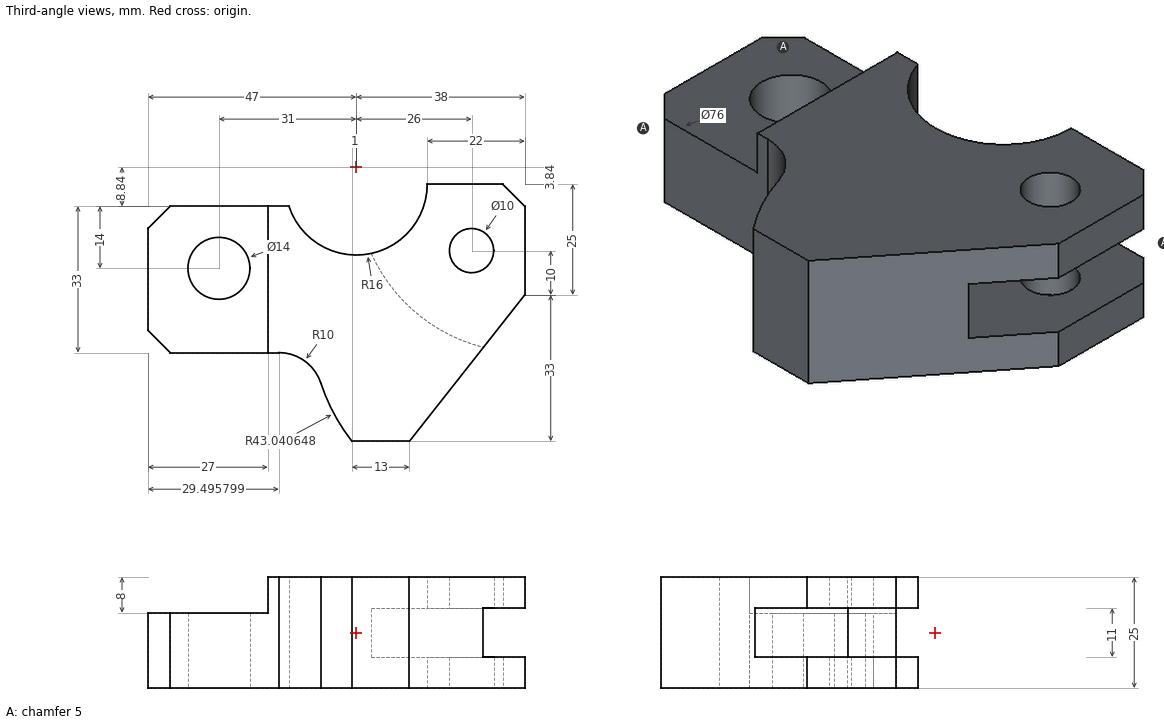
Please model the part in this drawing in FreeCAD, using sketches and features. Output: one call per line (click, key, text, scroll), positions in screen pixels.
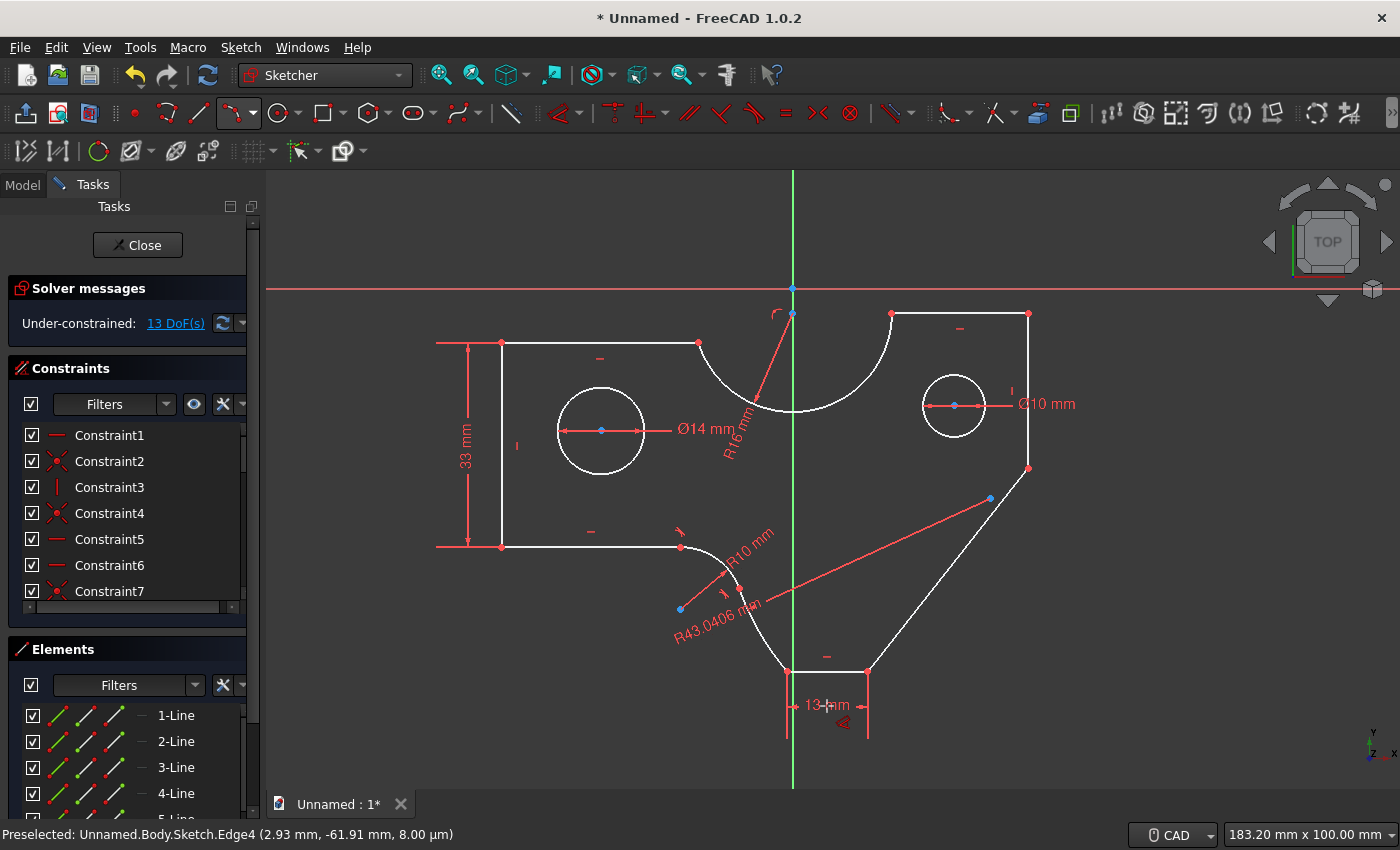
click(1028, 422)
click(1062, 391)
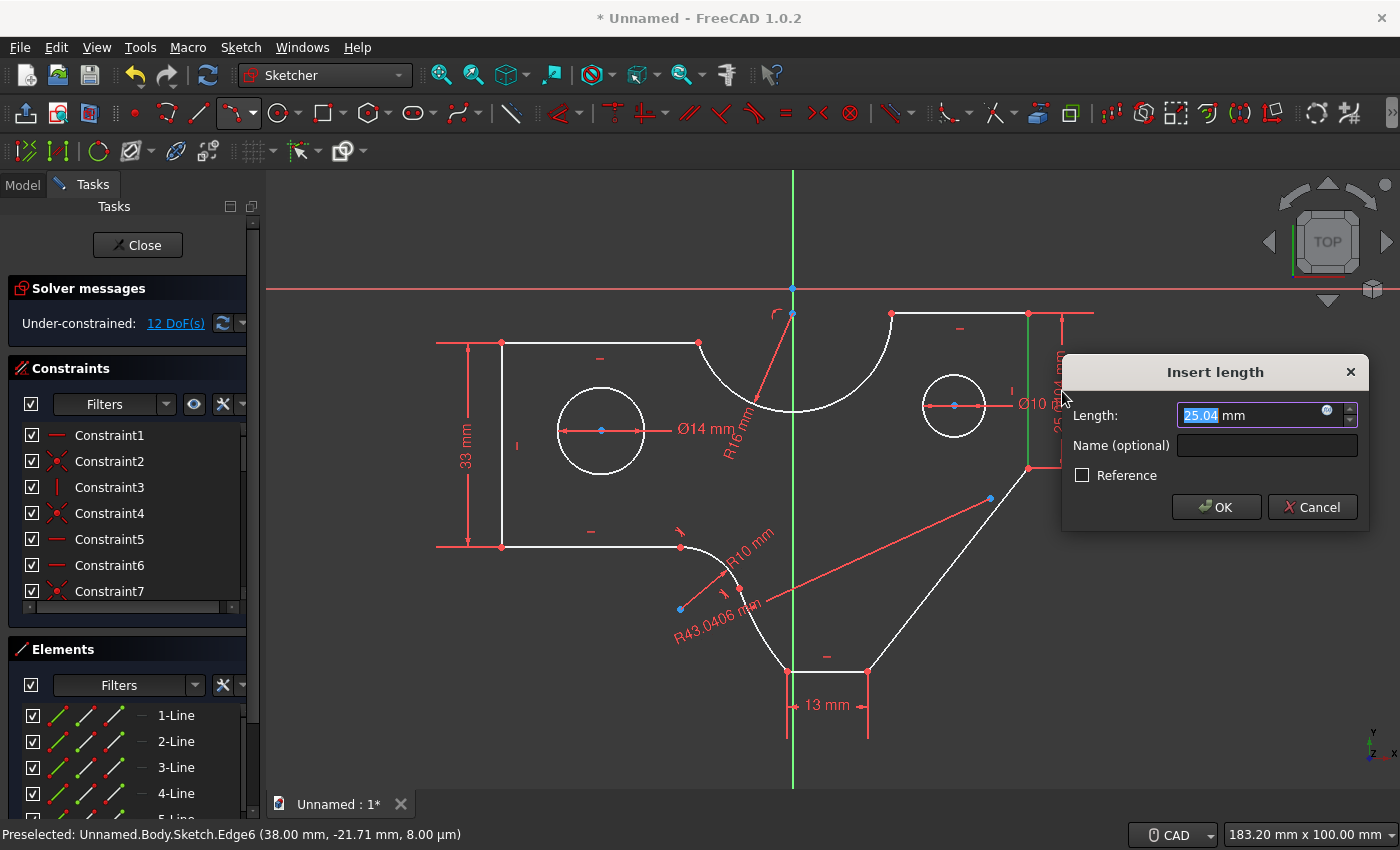
text(25)
key(Return)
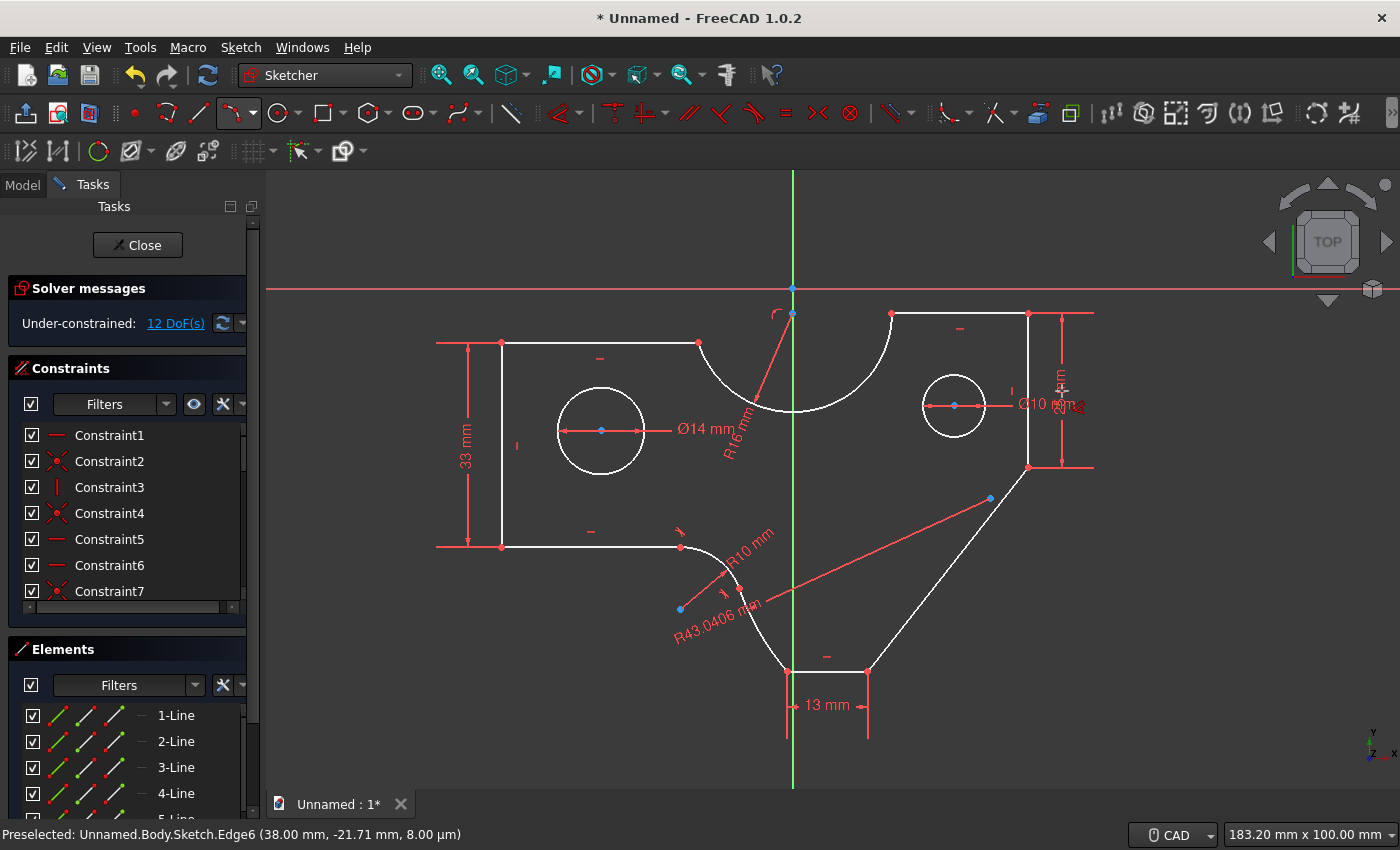
click(987, 313)
click(960, 347)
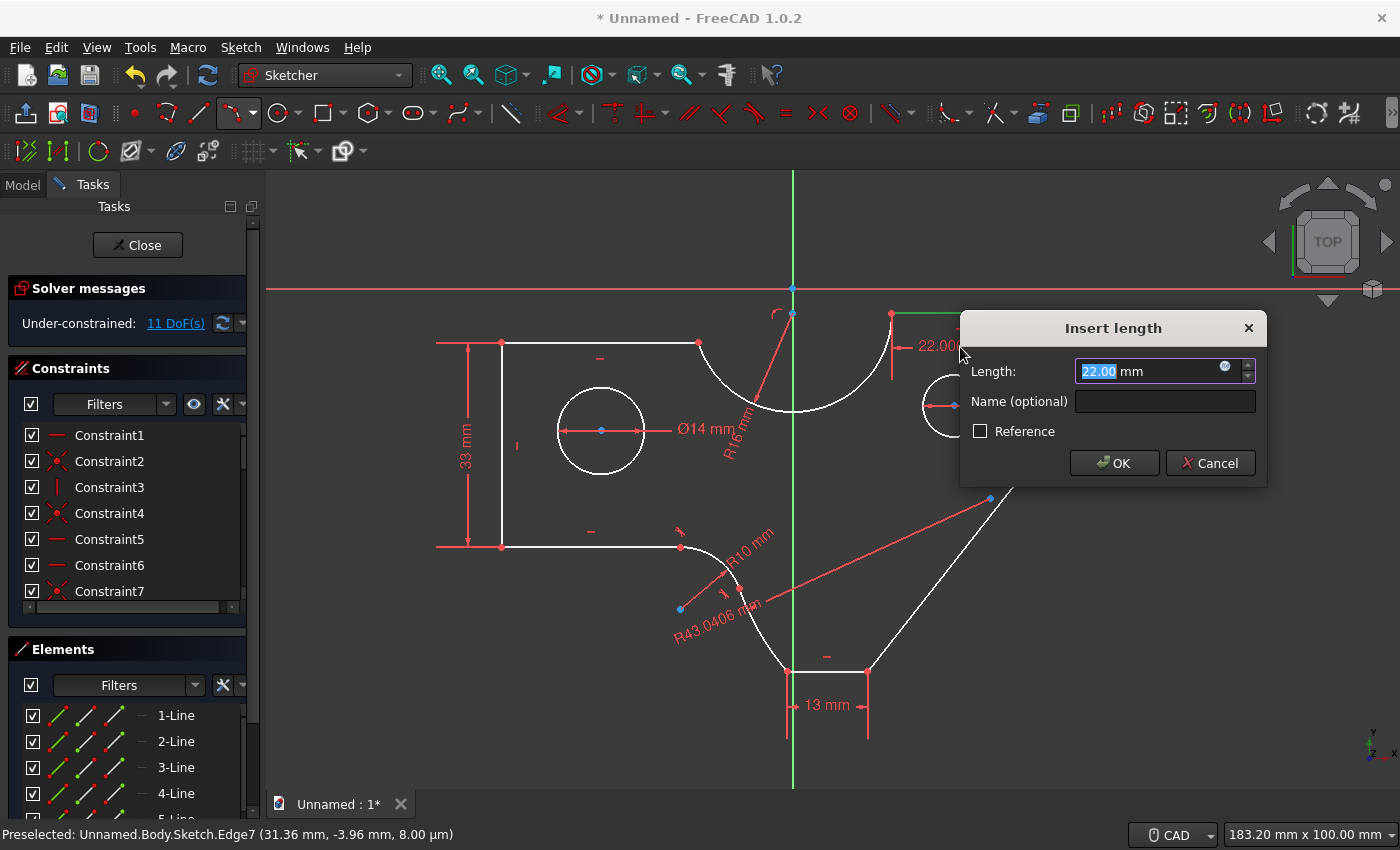
text(22)
key(Return)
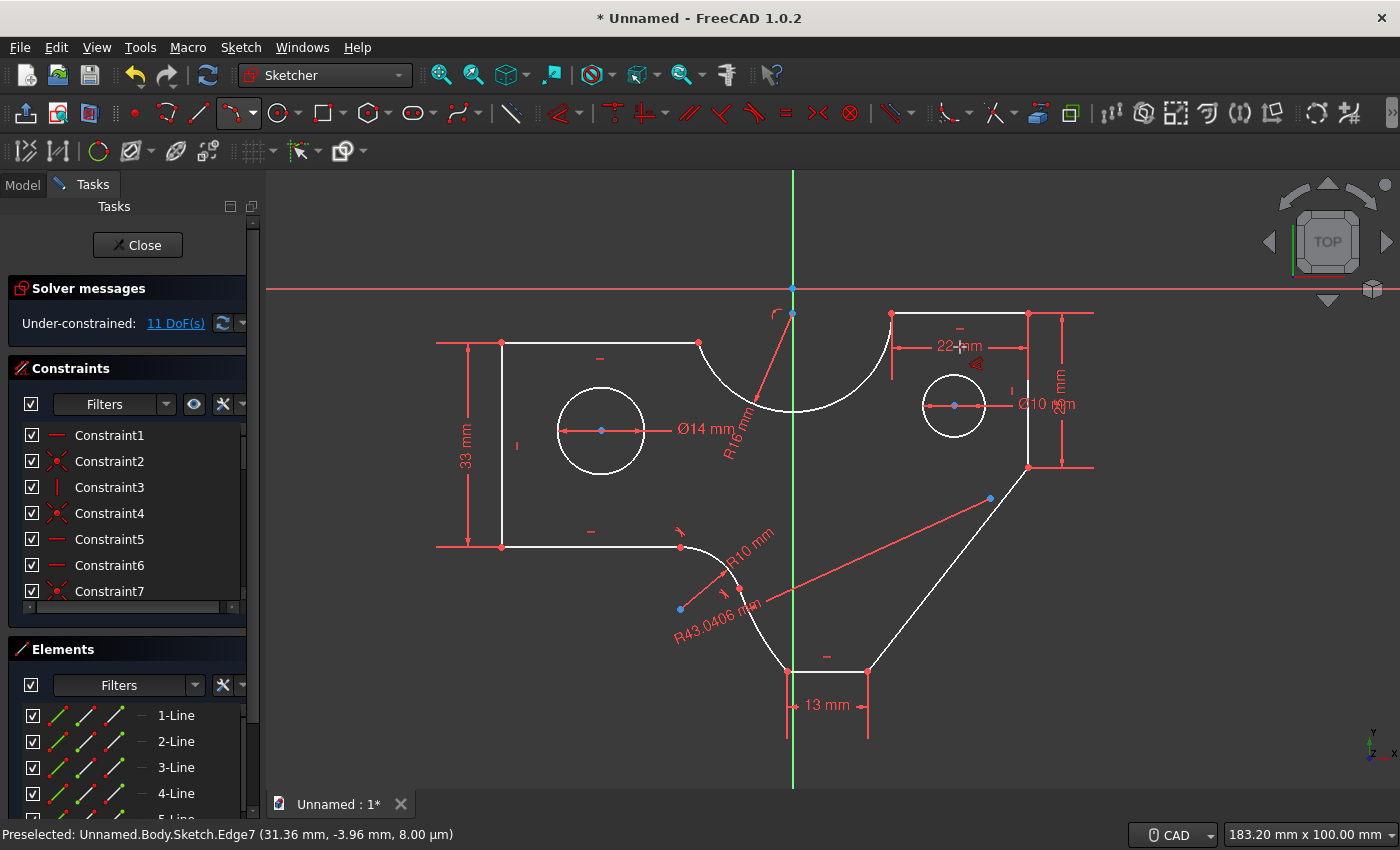
scroll(787, 672, up, 10)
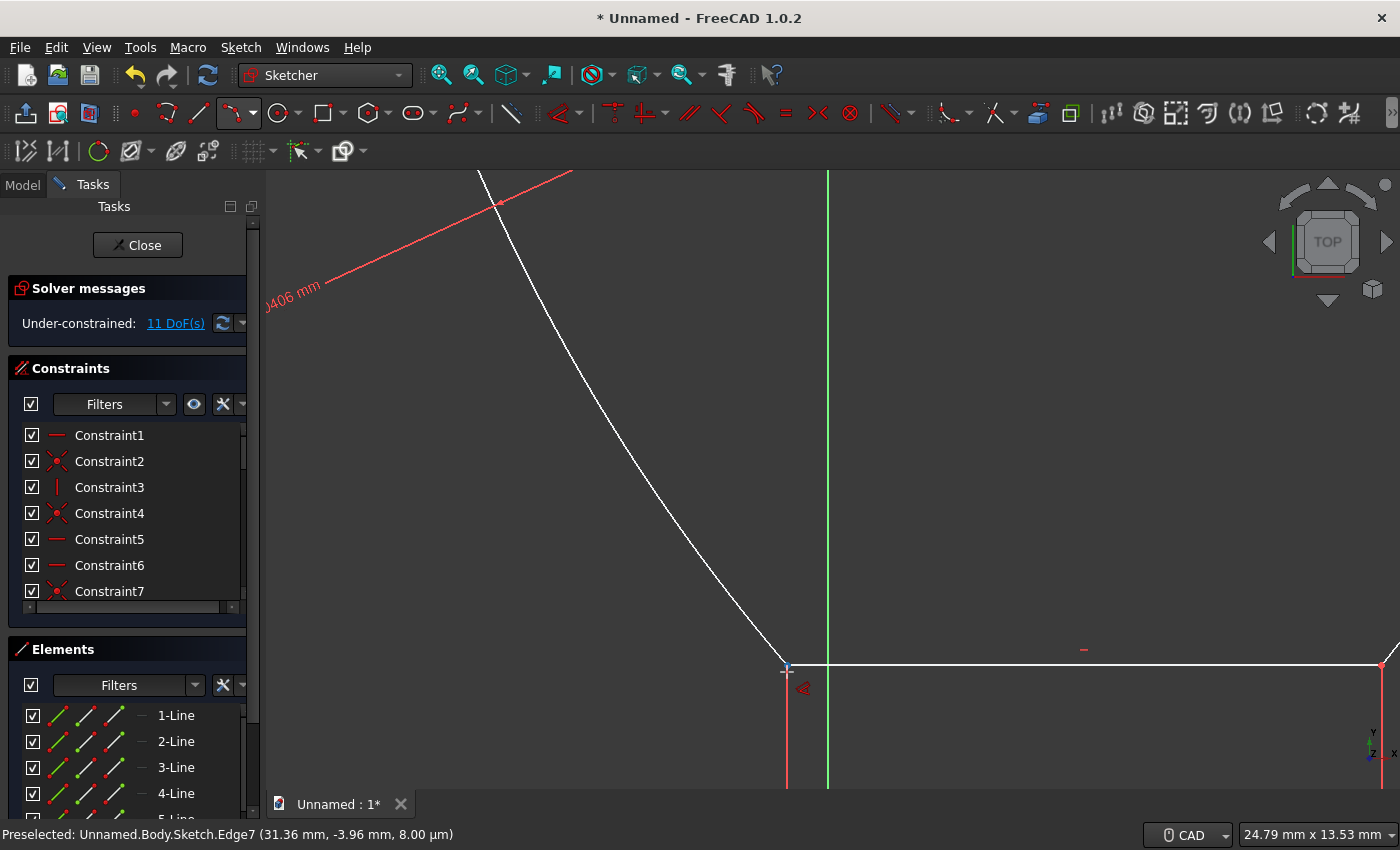
click(787, 665)
click(807, 699)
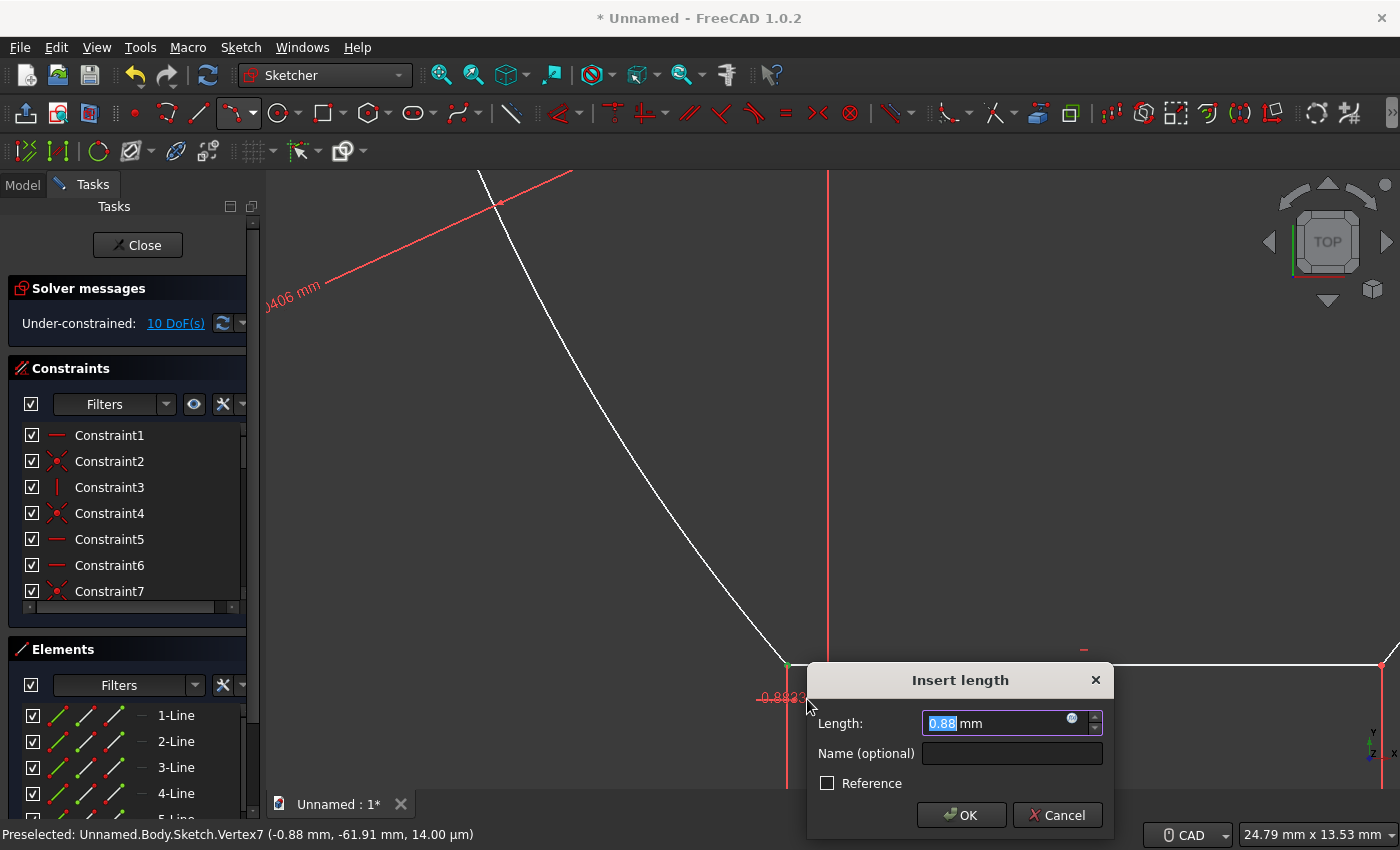
text(1)
key(Return)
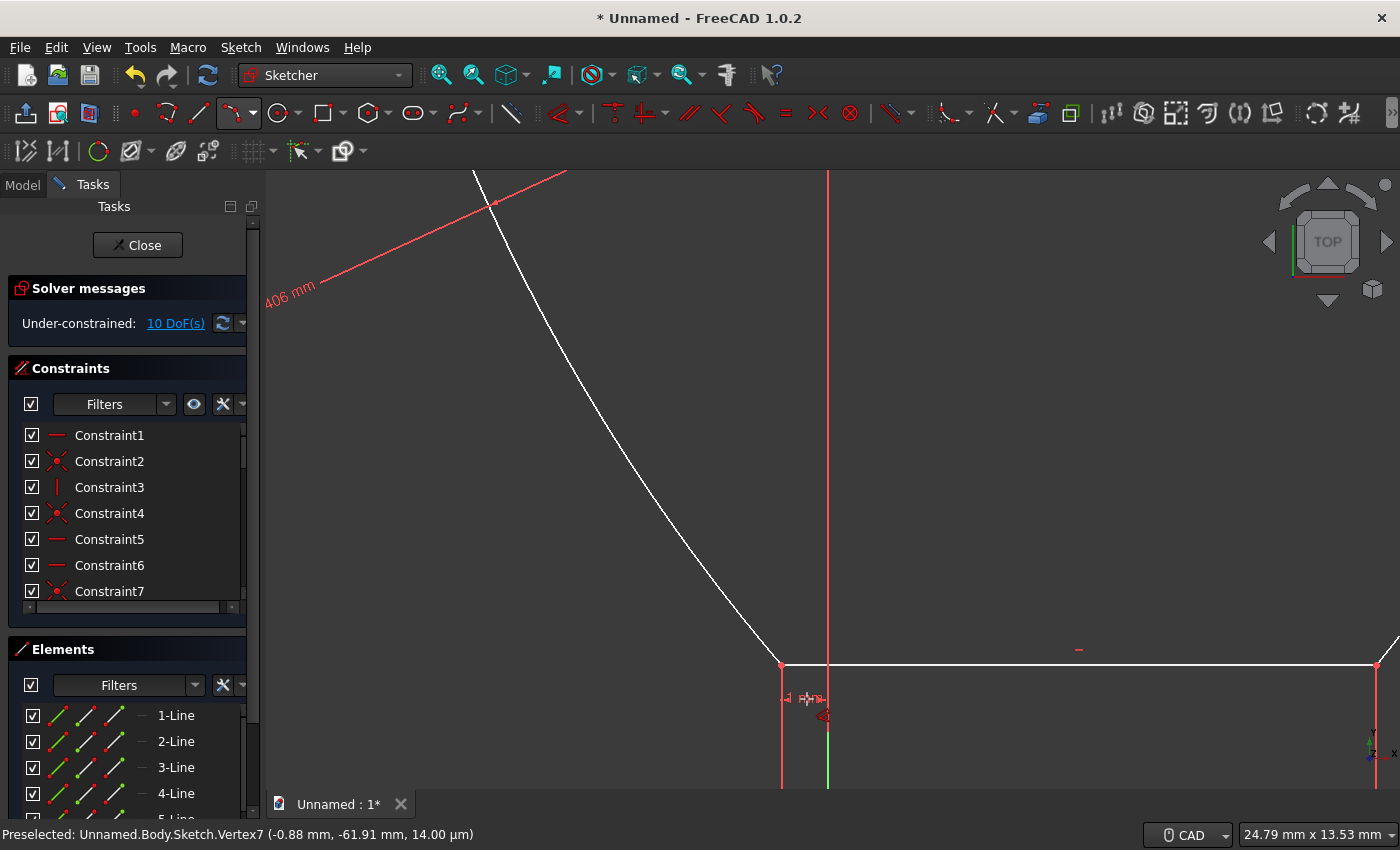
scroll(787, 672, down, 10)